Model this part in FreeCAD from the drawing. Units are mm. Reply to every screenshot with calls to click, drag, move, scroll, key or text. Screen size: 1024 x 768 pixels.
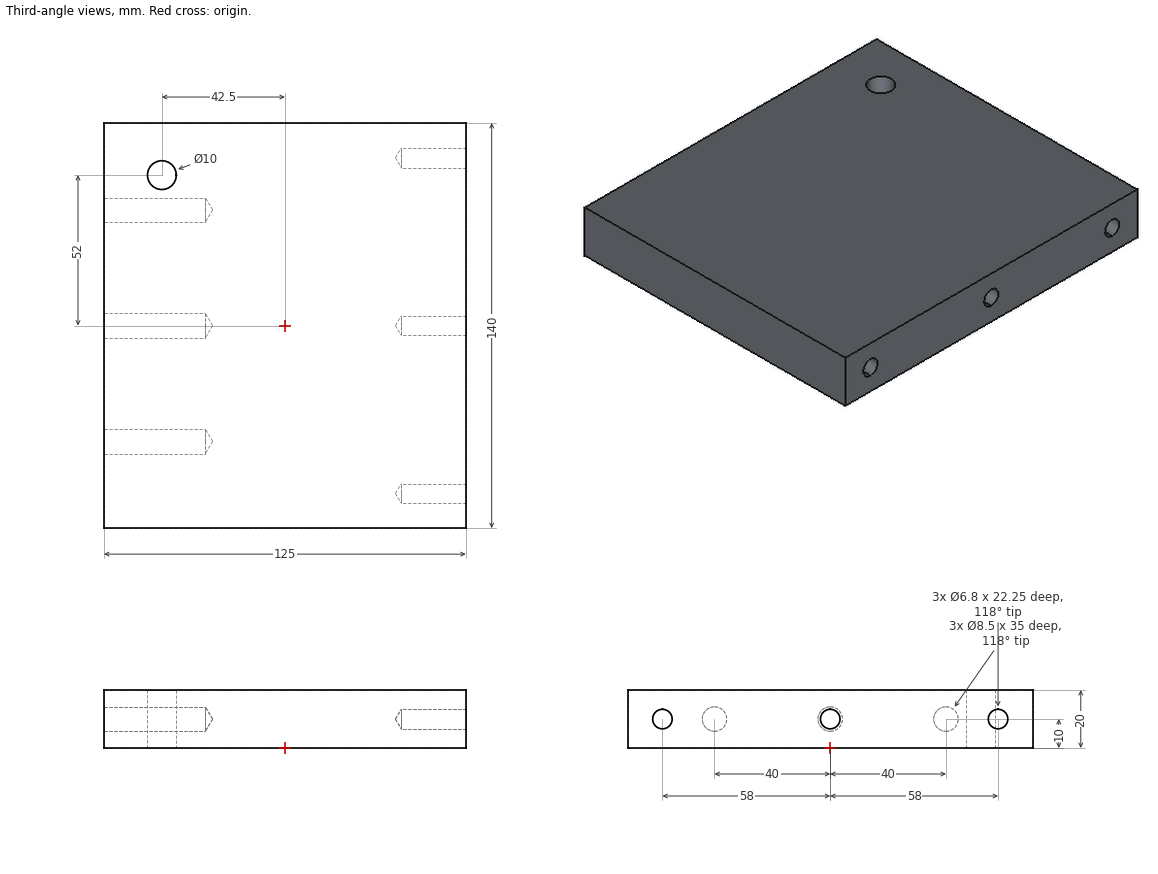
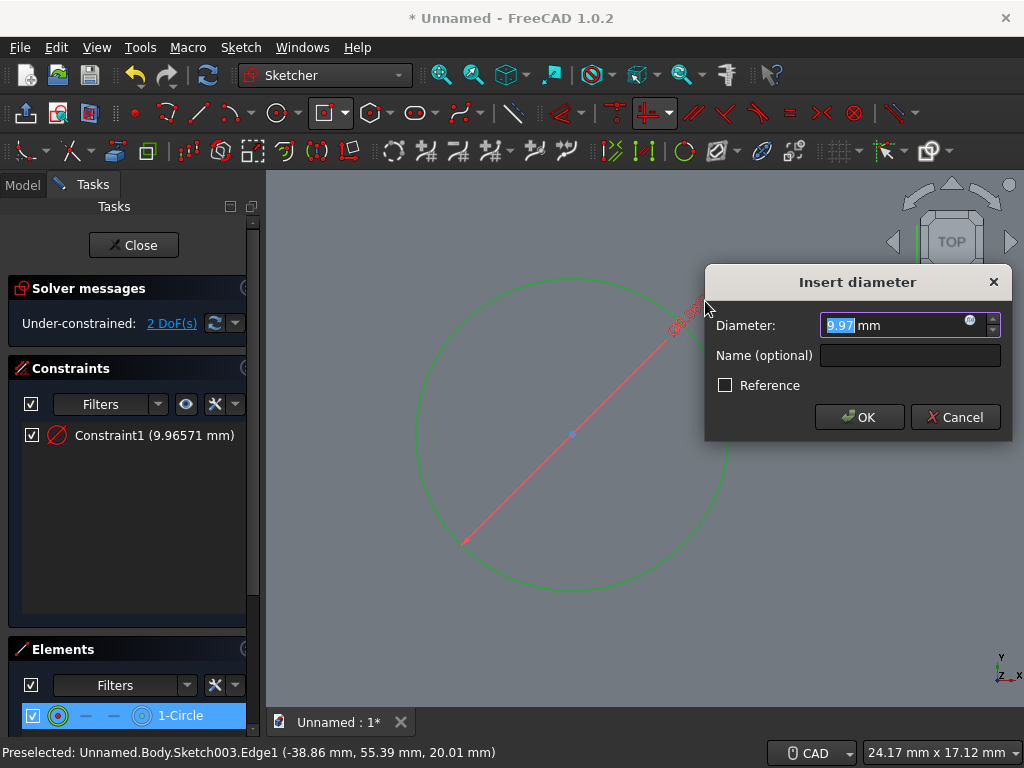
text(10)
key(Return)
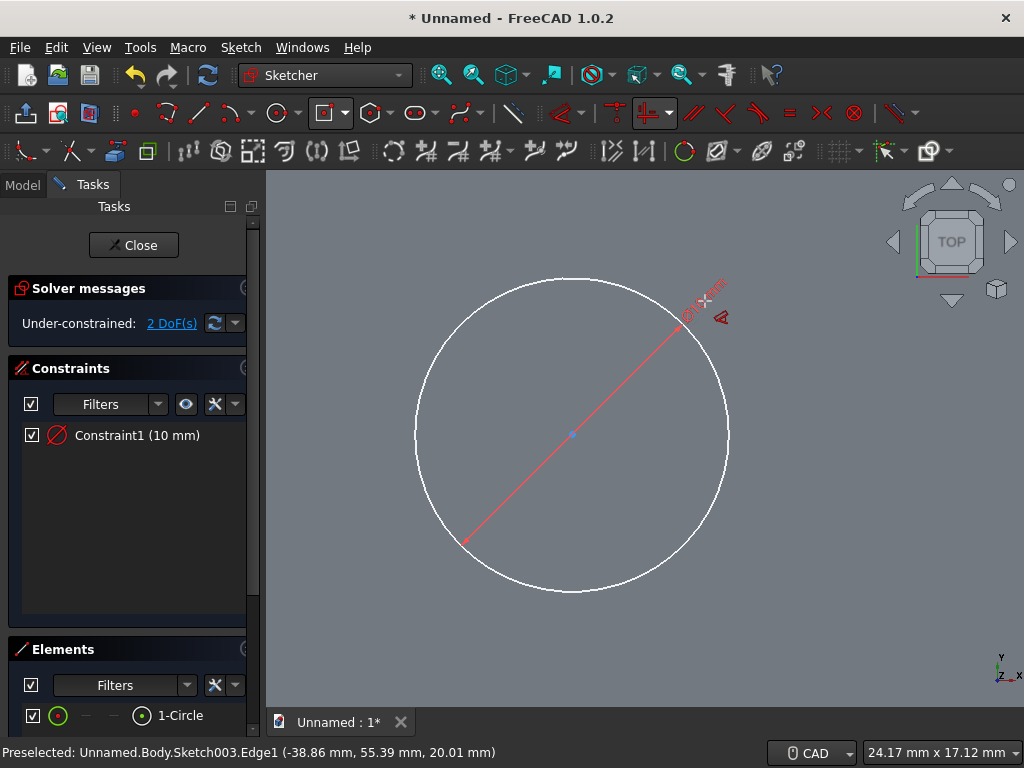
click(572, 435)
click(538, 557)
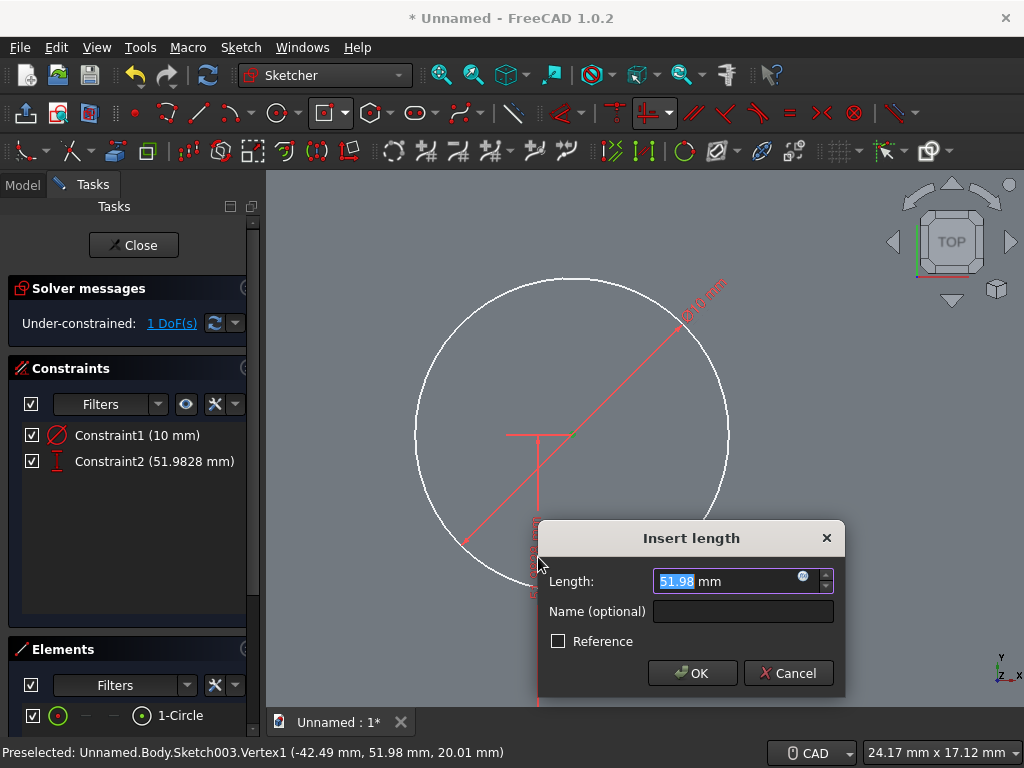
text(52)
key(Return)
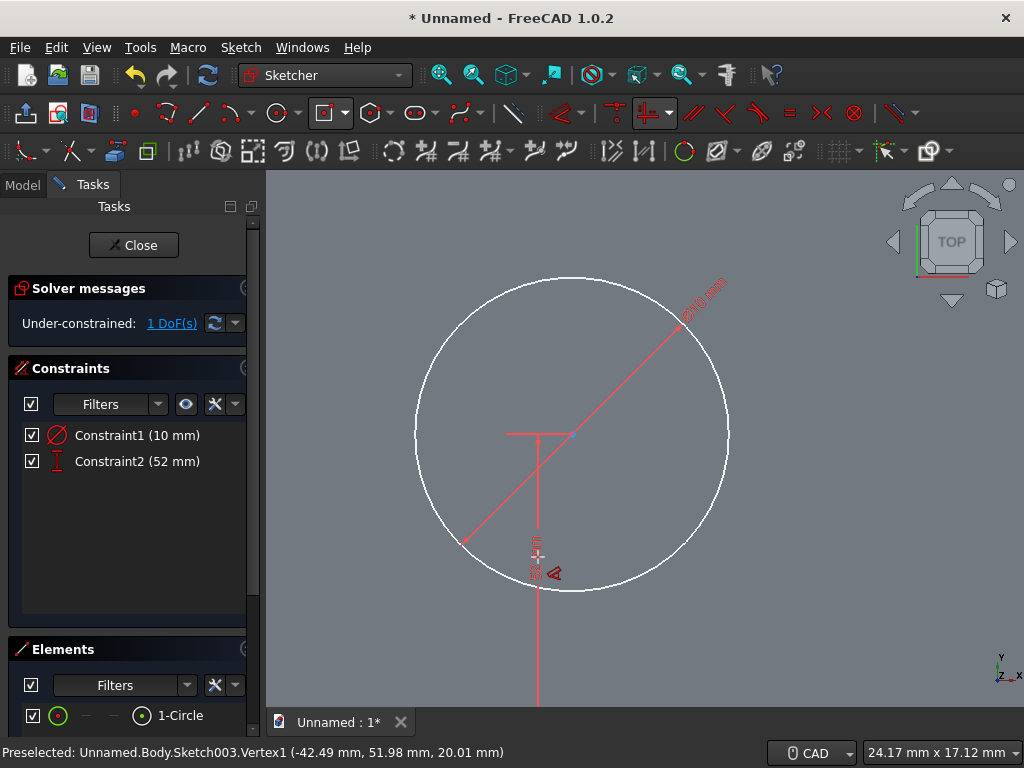
click(572, 434)
click(649, 400)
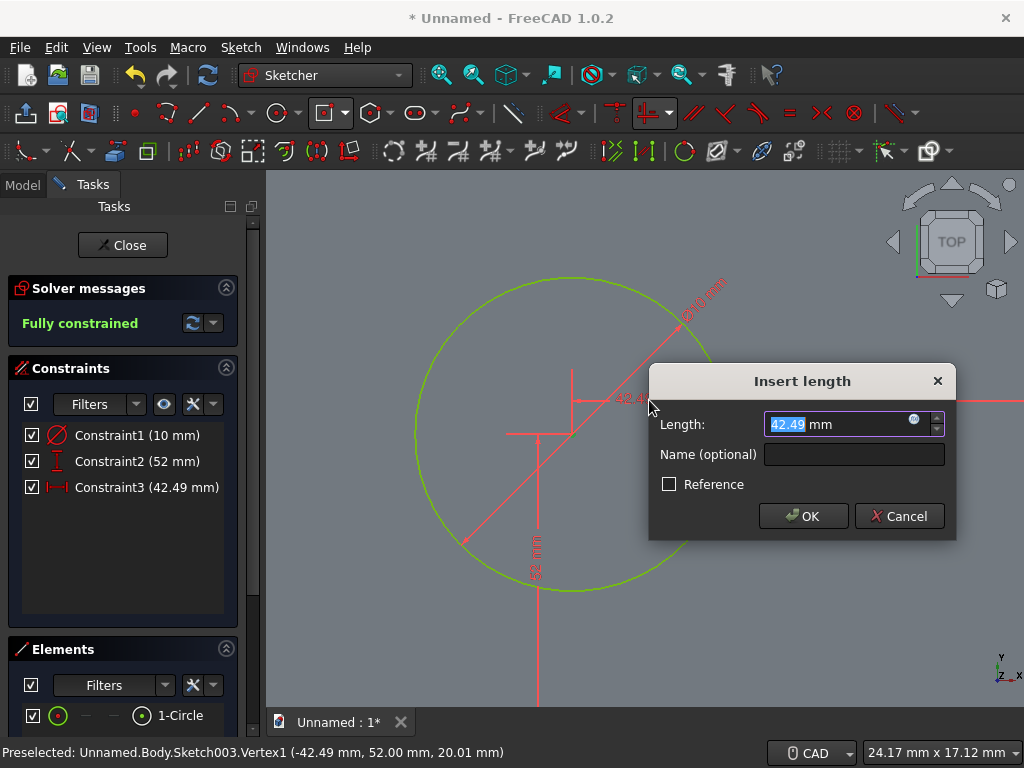
text(42.5)
key(Return)
key(Escape)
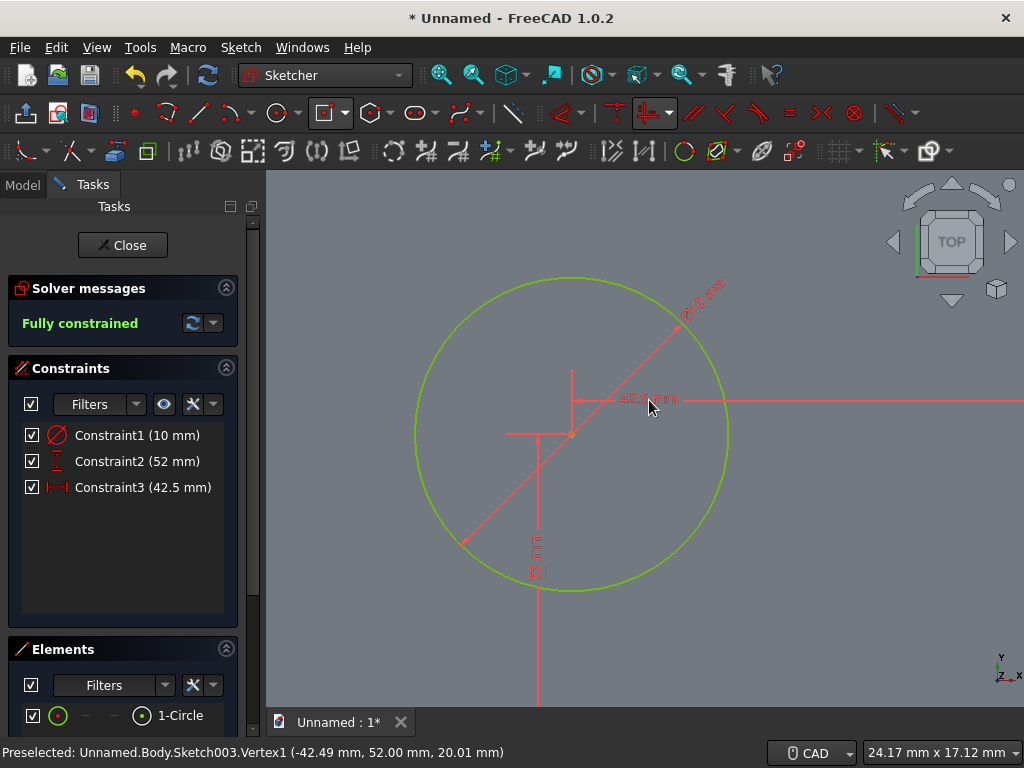
click(123, 245)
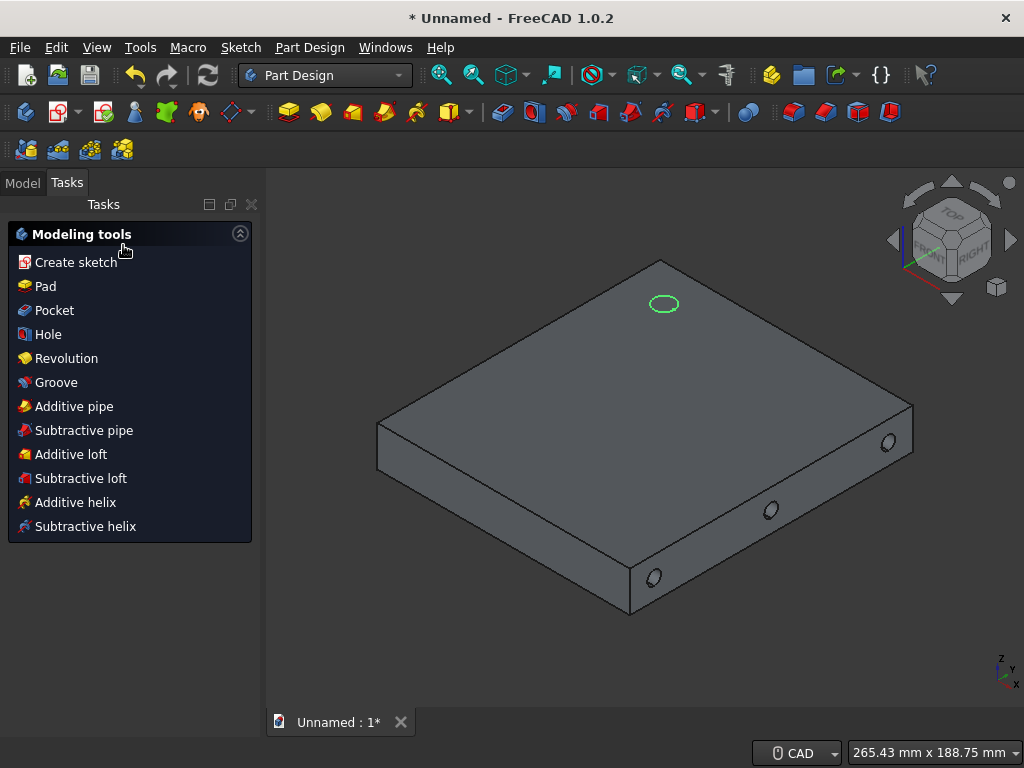
click(504, 112)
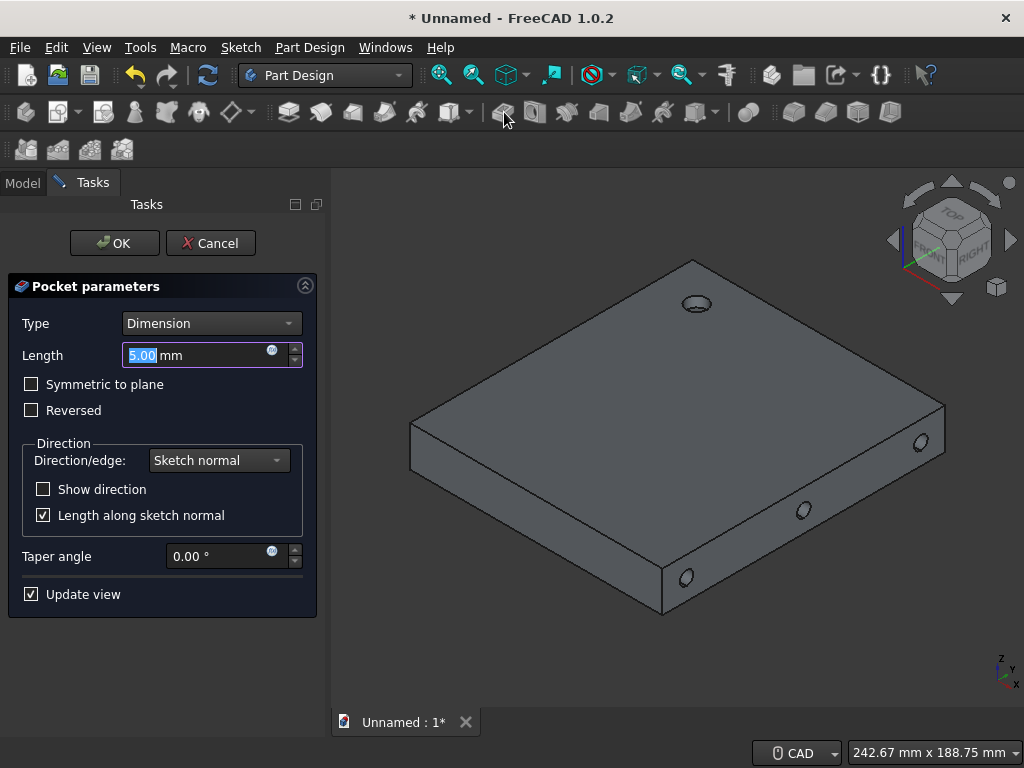
click(212, 324)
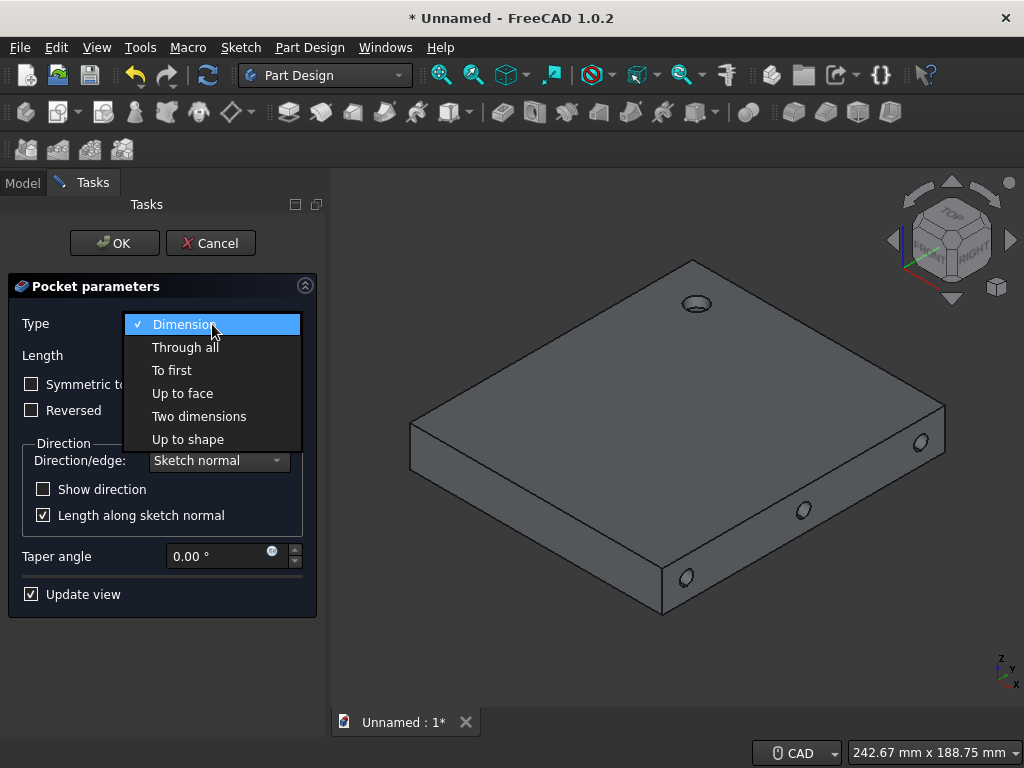
click(212, 348)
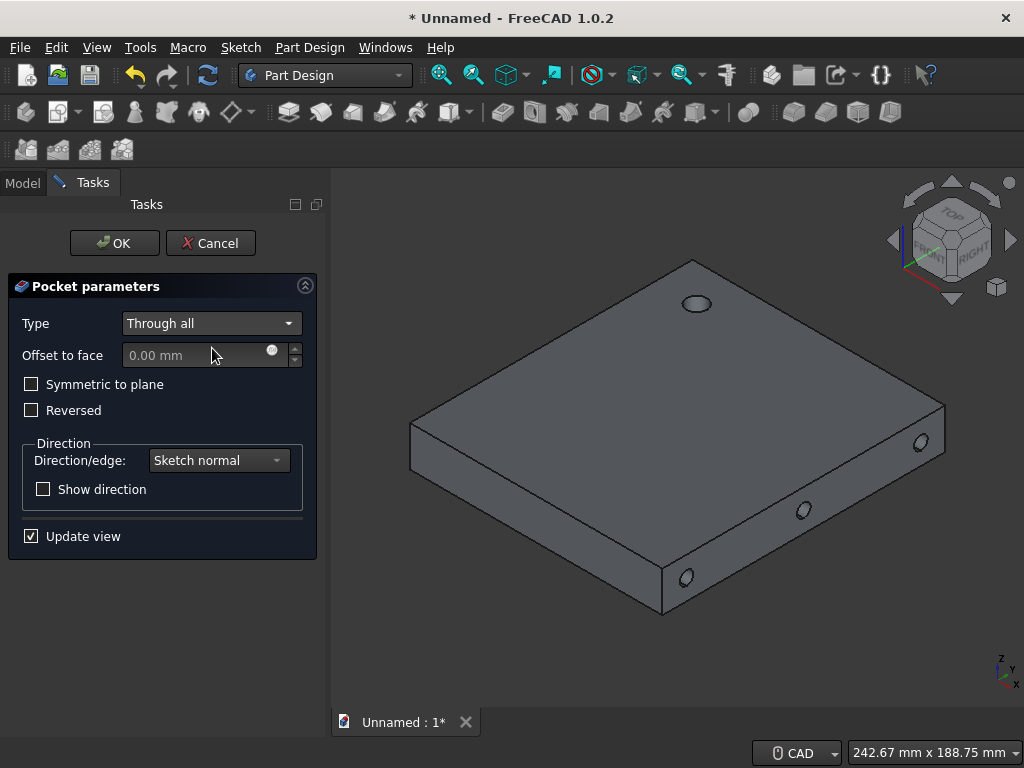
click(115, 243)